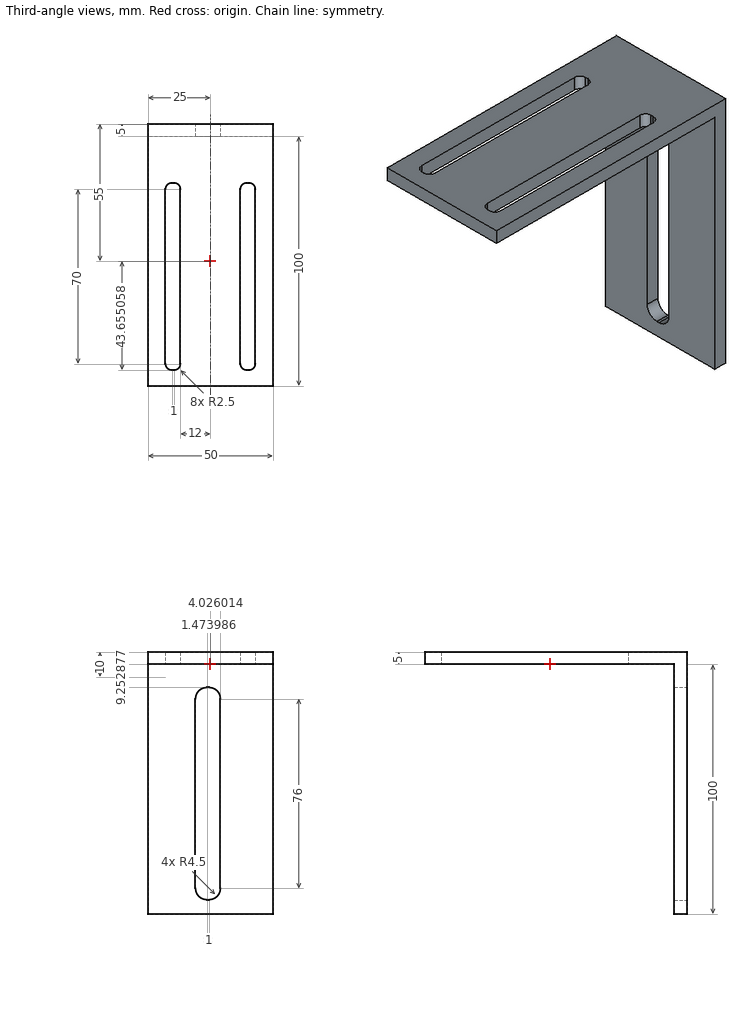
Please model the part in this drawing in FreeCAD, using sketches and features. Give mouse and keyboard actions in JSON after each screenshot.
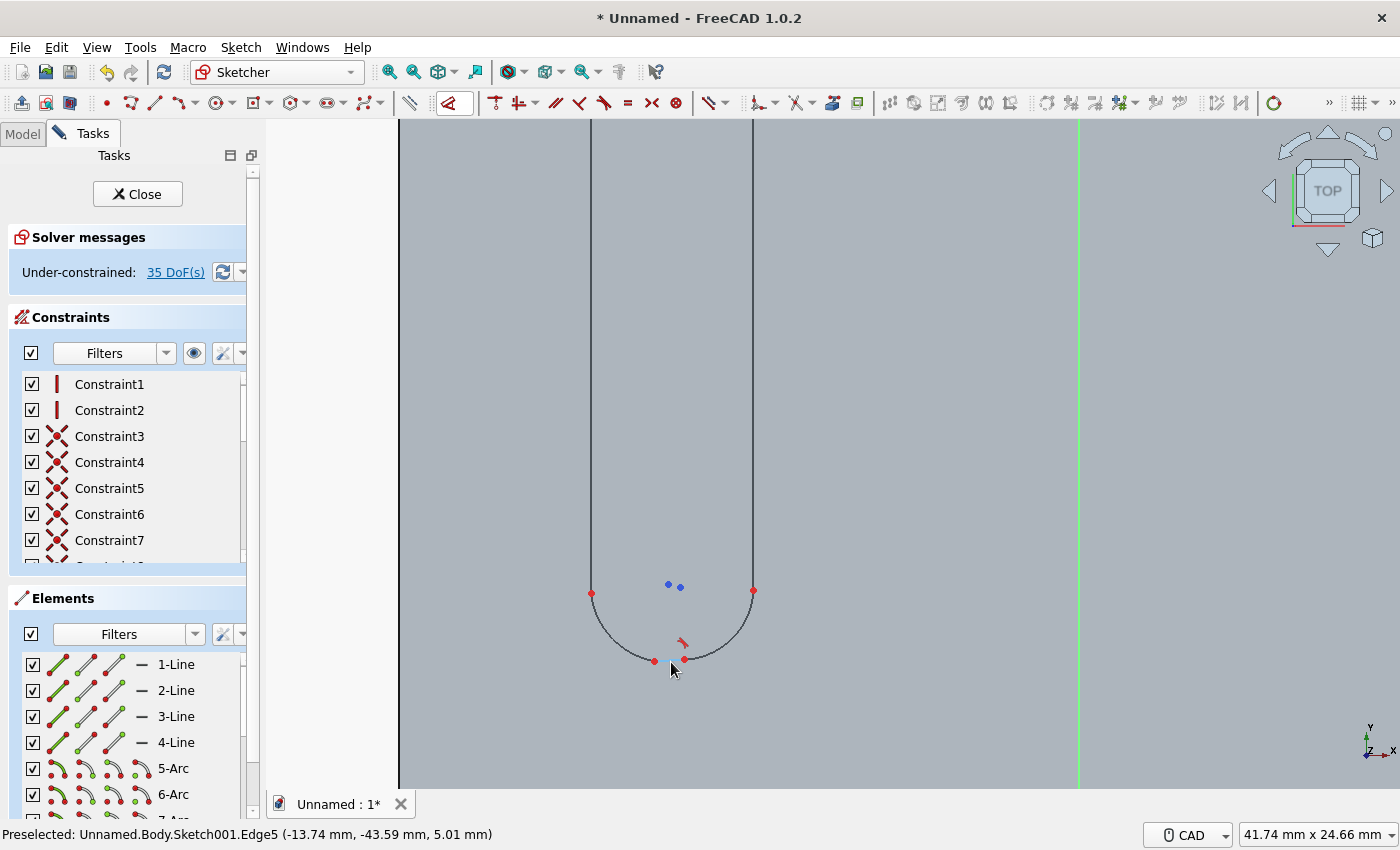
{"action": "left_click", "coordinate": [670, 660]}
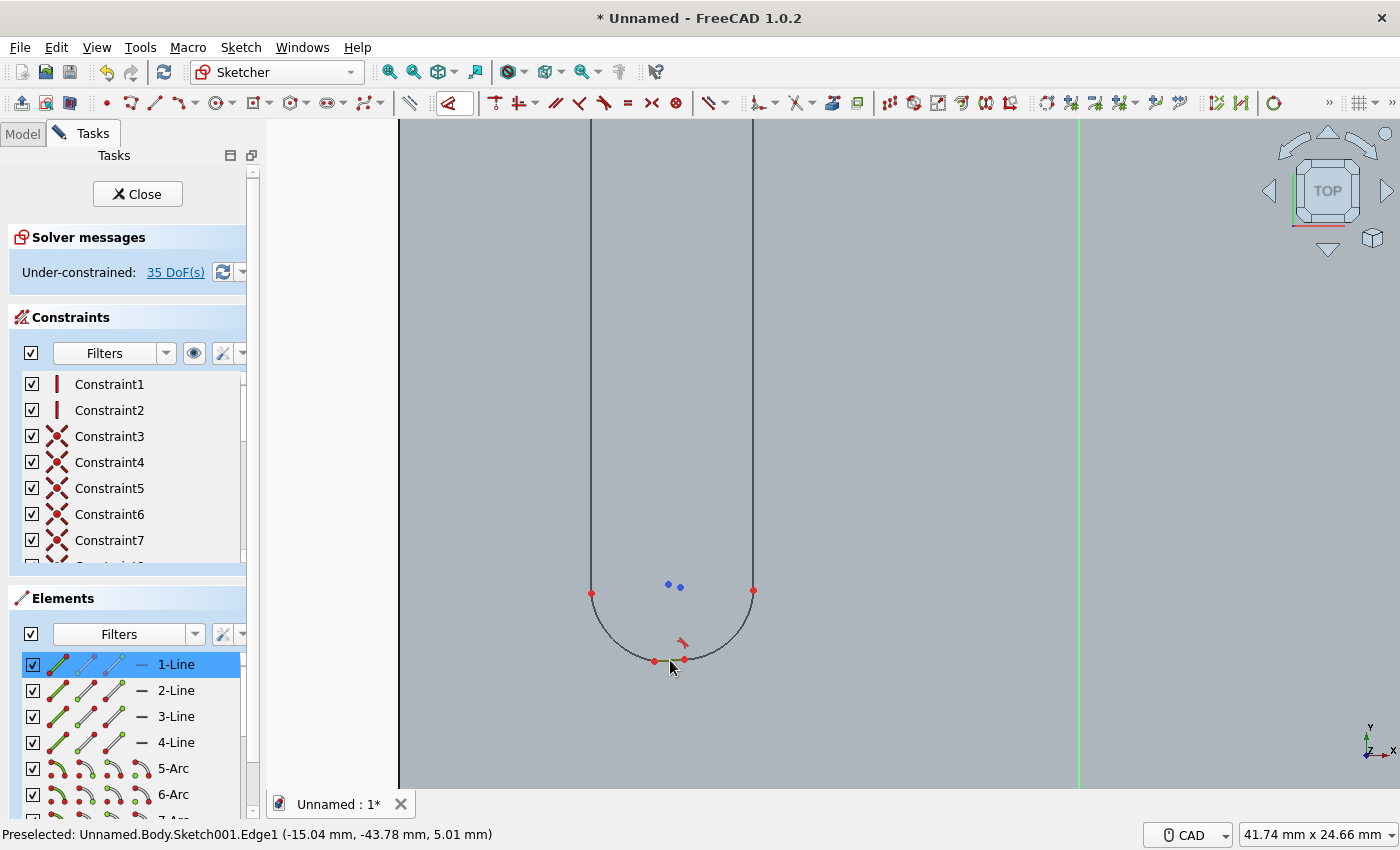
{"action": "left_click", "coordinate": [600, 622]}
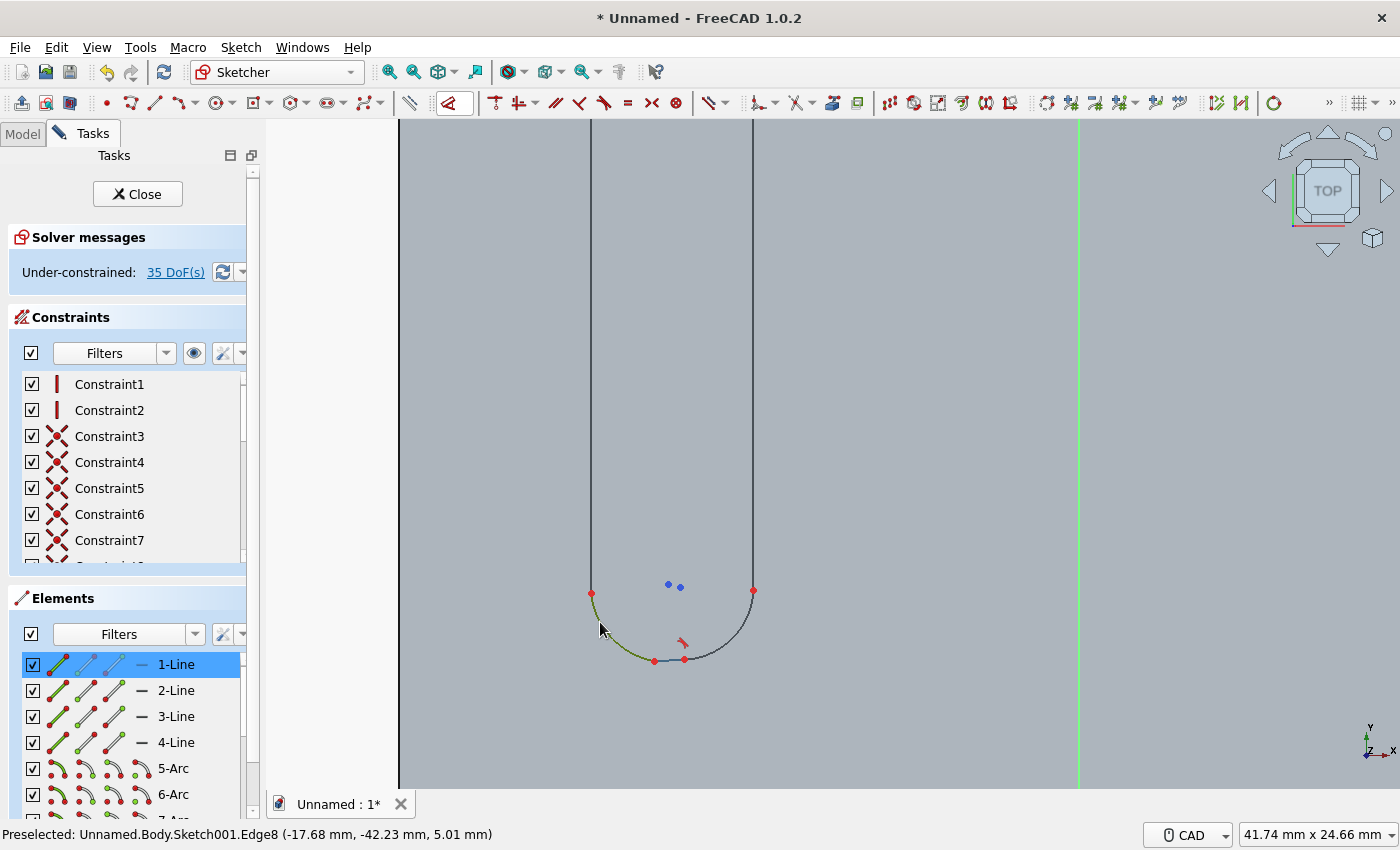
{"action": "key", "text": "t"}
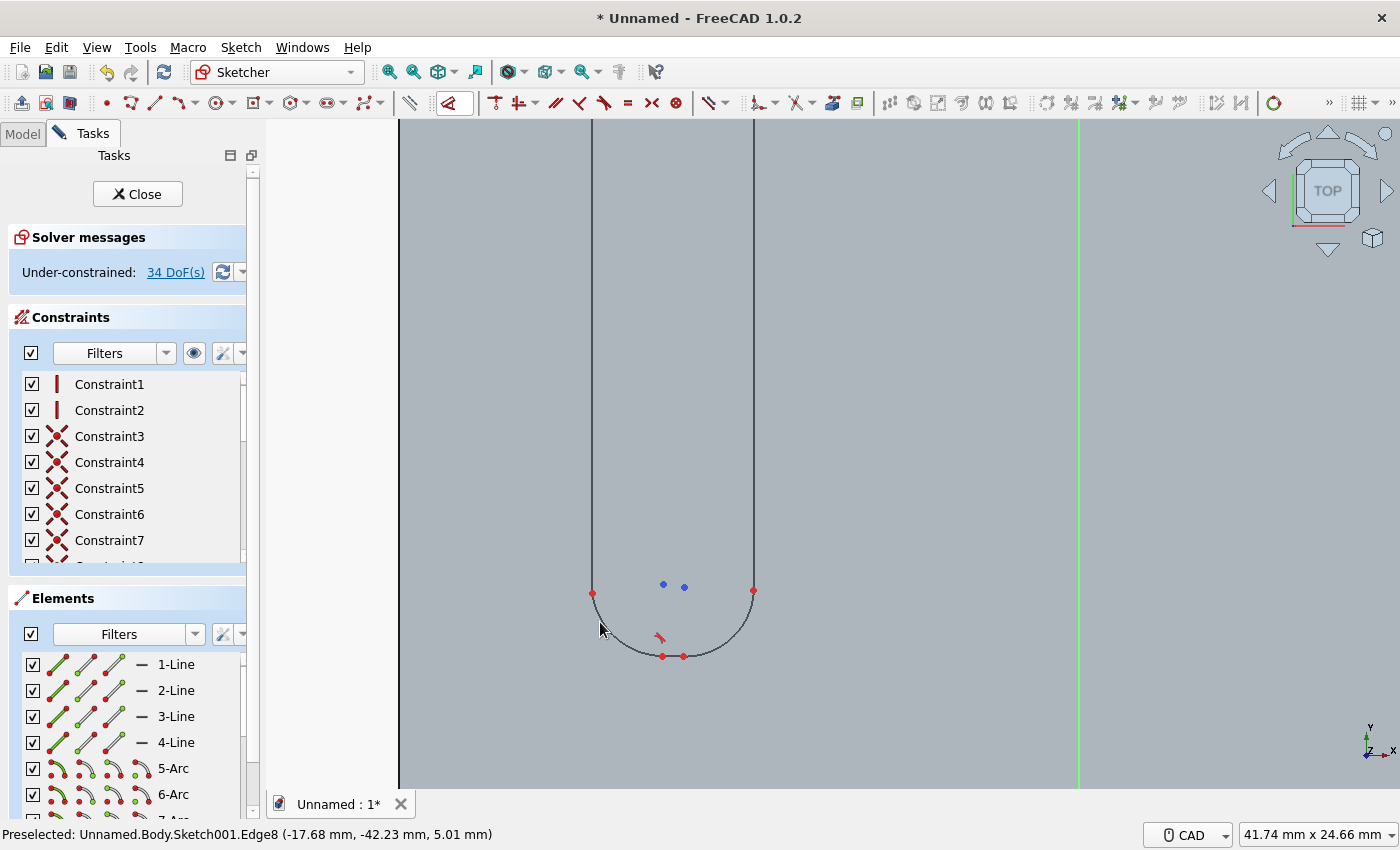
{"action": "scroll", "coordinate": [685, 660], "scroll_direction": "down", "scroll_amount": 8}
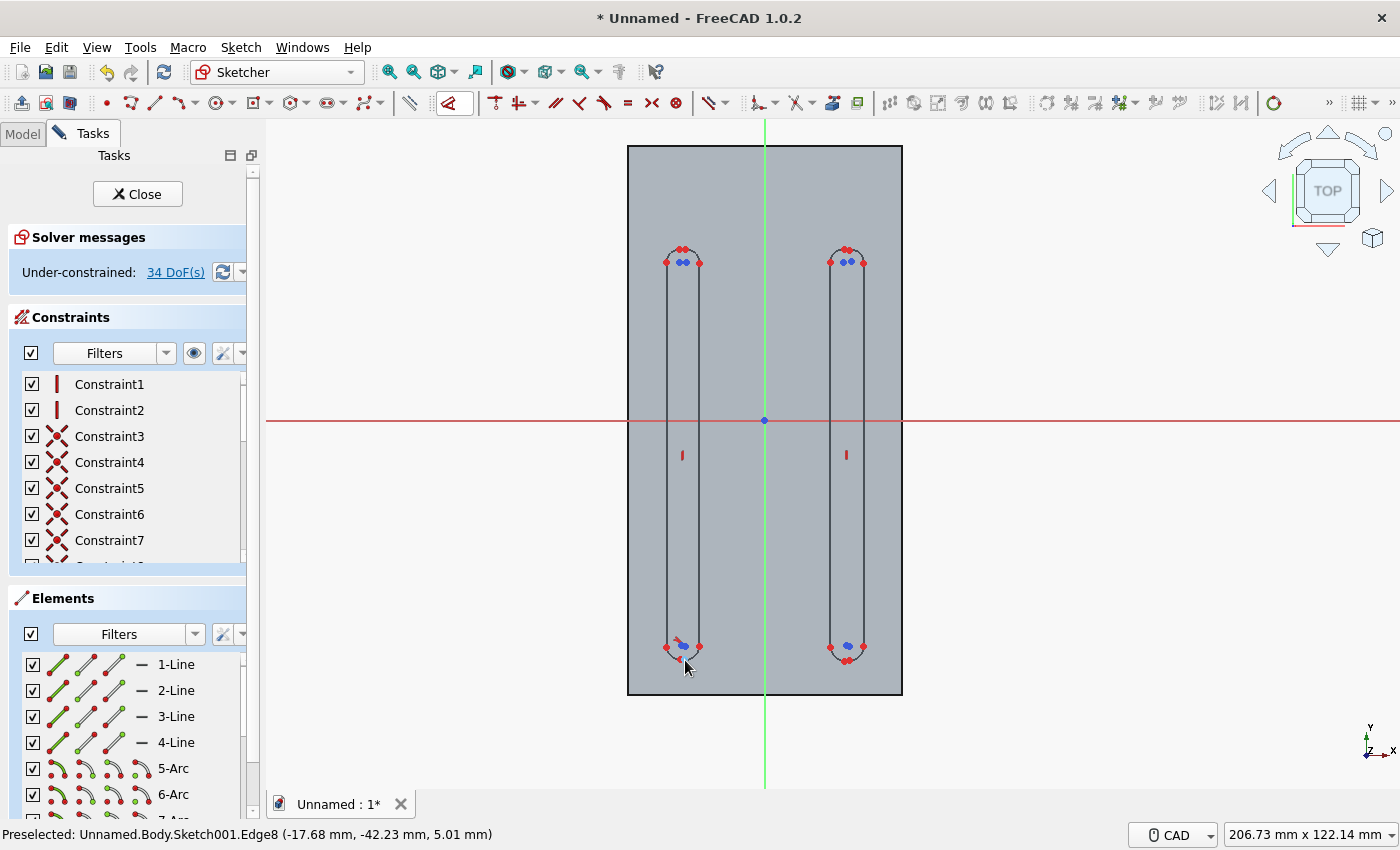
{"action": "left_click", "coordinate": [699, 570]}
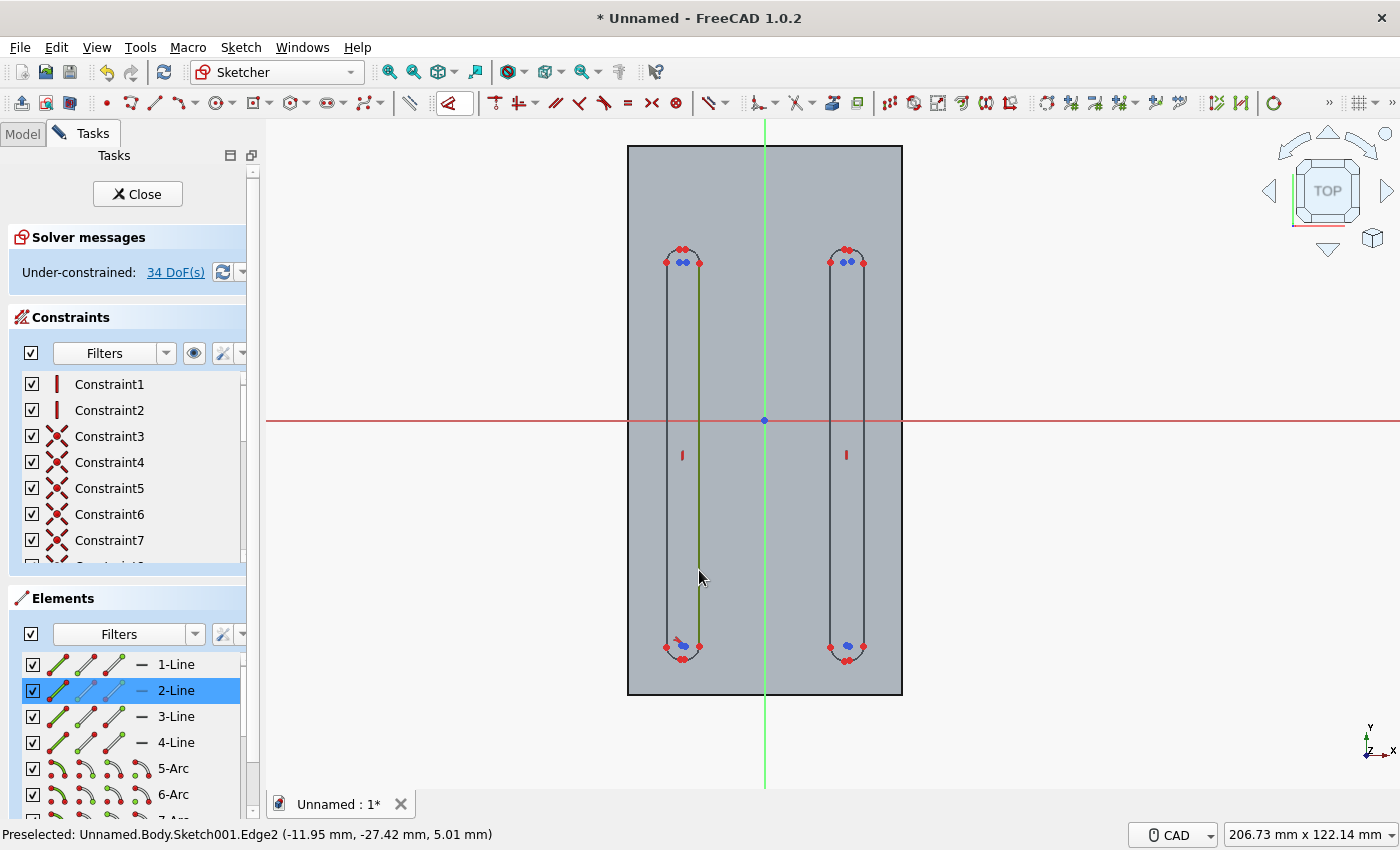
{"action": "scroll", "coordinate": [695, 656], "scroll_direction": "up", "scroll_amount": 2}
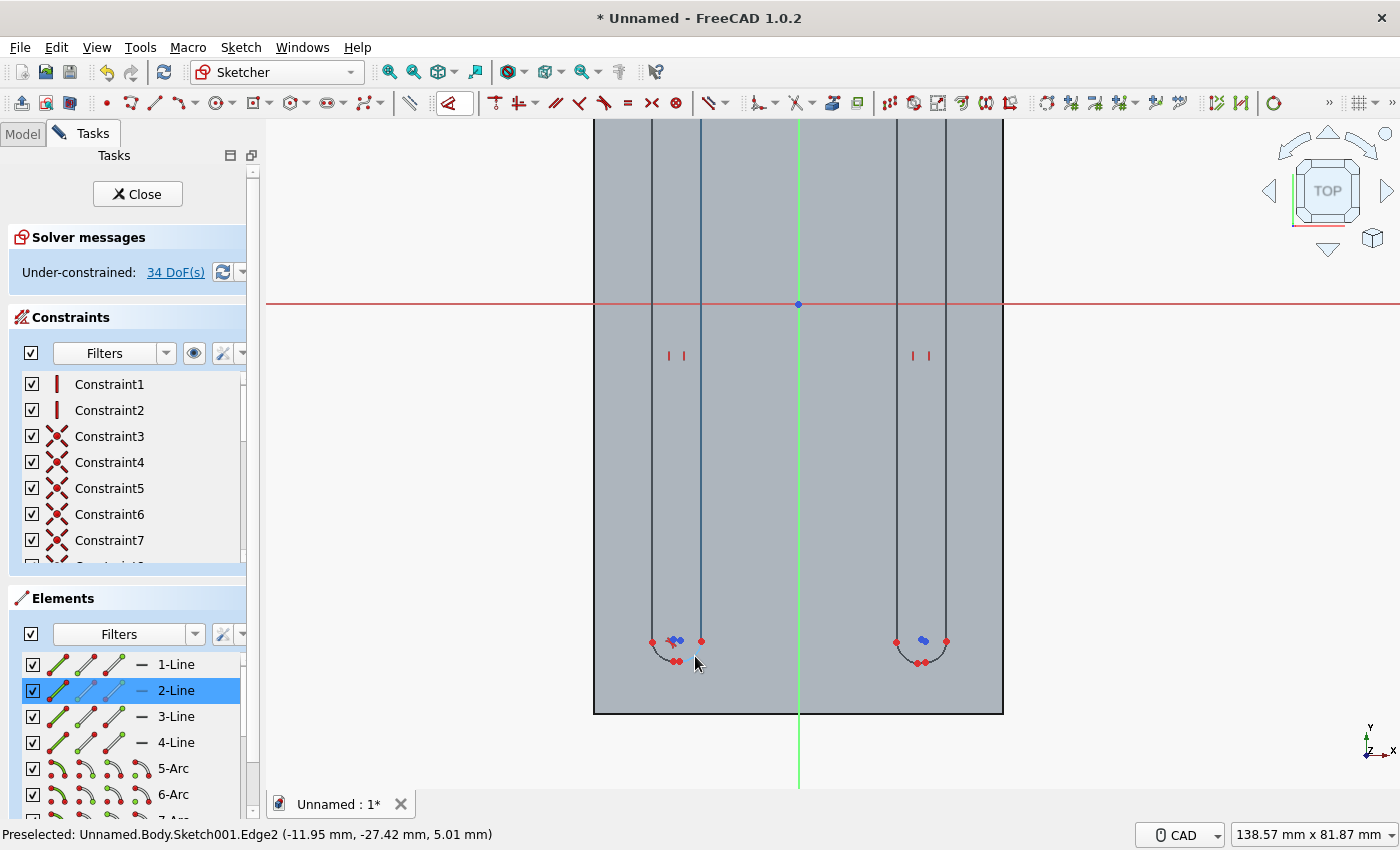
{"action": "left_click", "coordinate": [694, 656]}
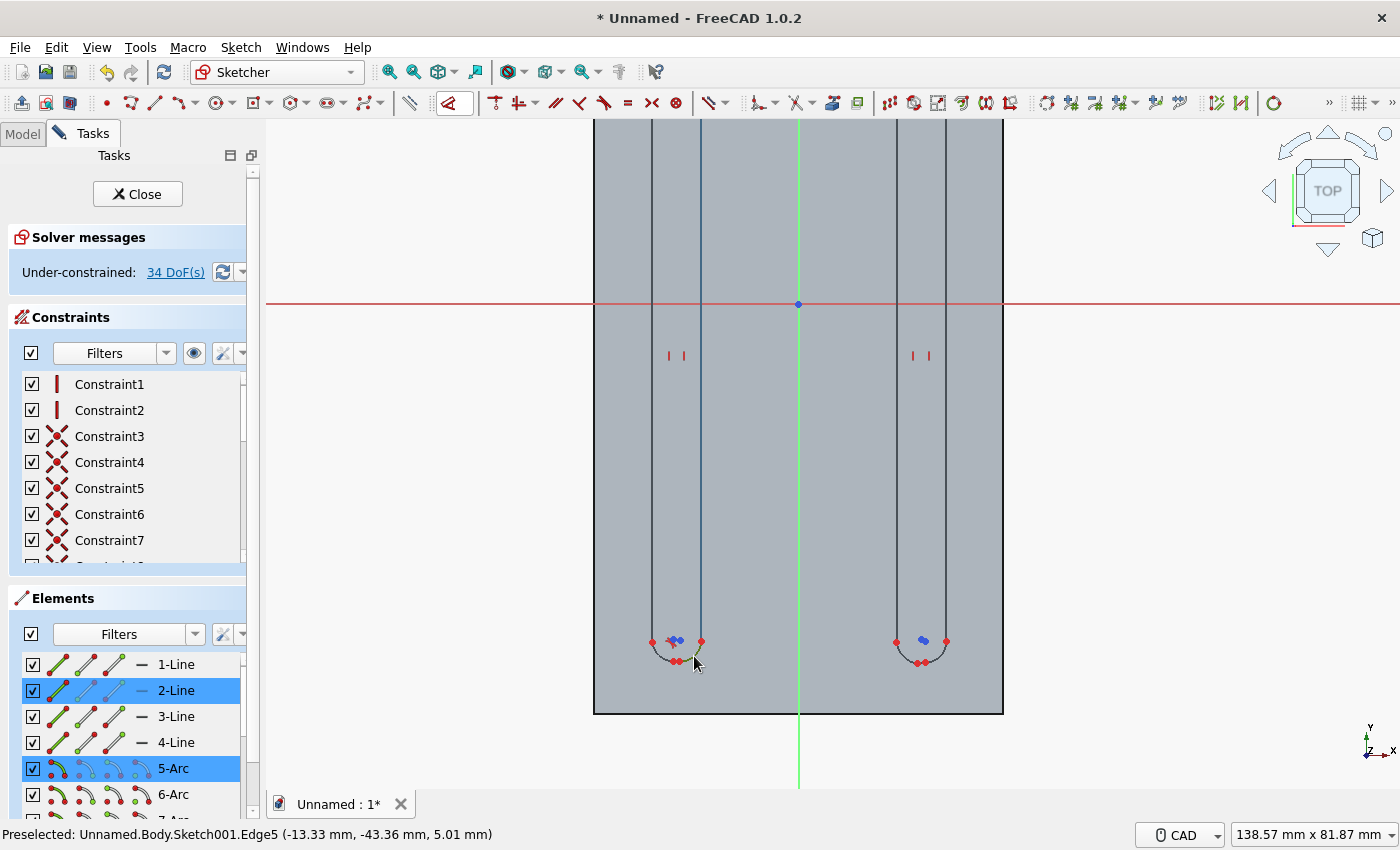
{"action": "key", "text": "t"}